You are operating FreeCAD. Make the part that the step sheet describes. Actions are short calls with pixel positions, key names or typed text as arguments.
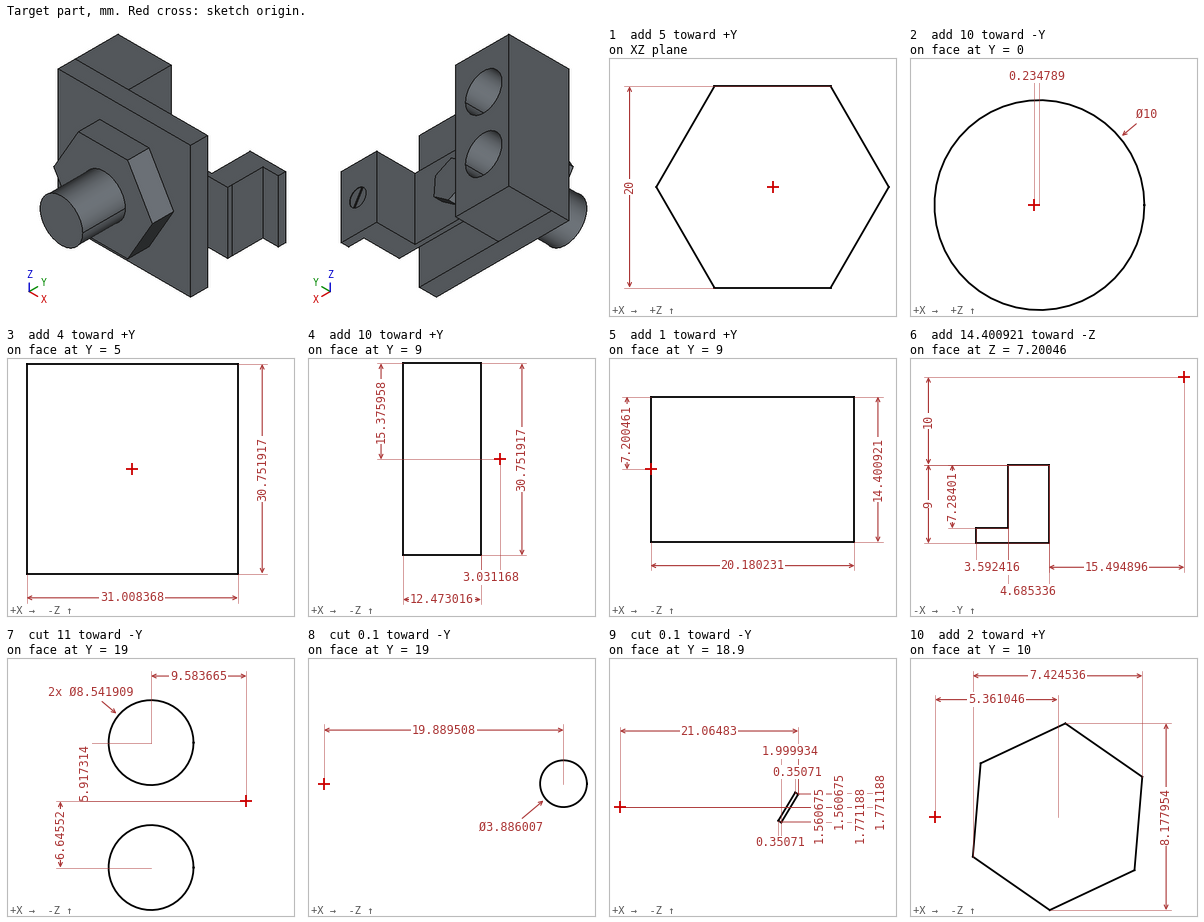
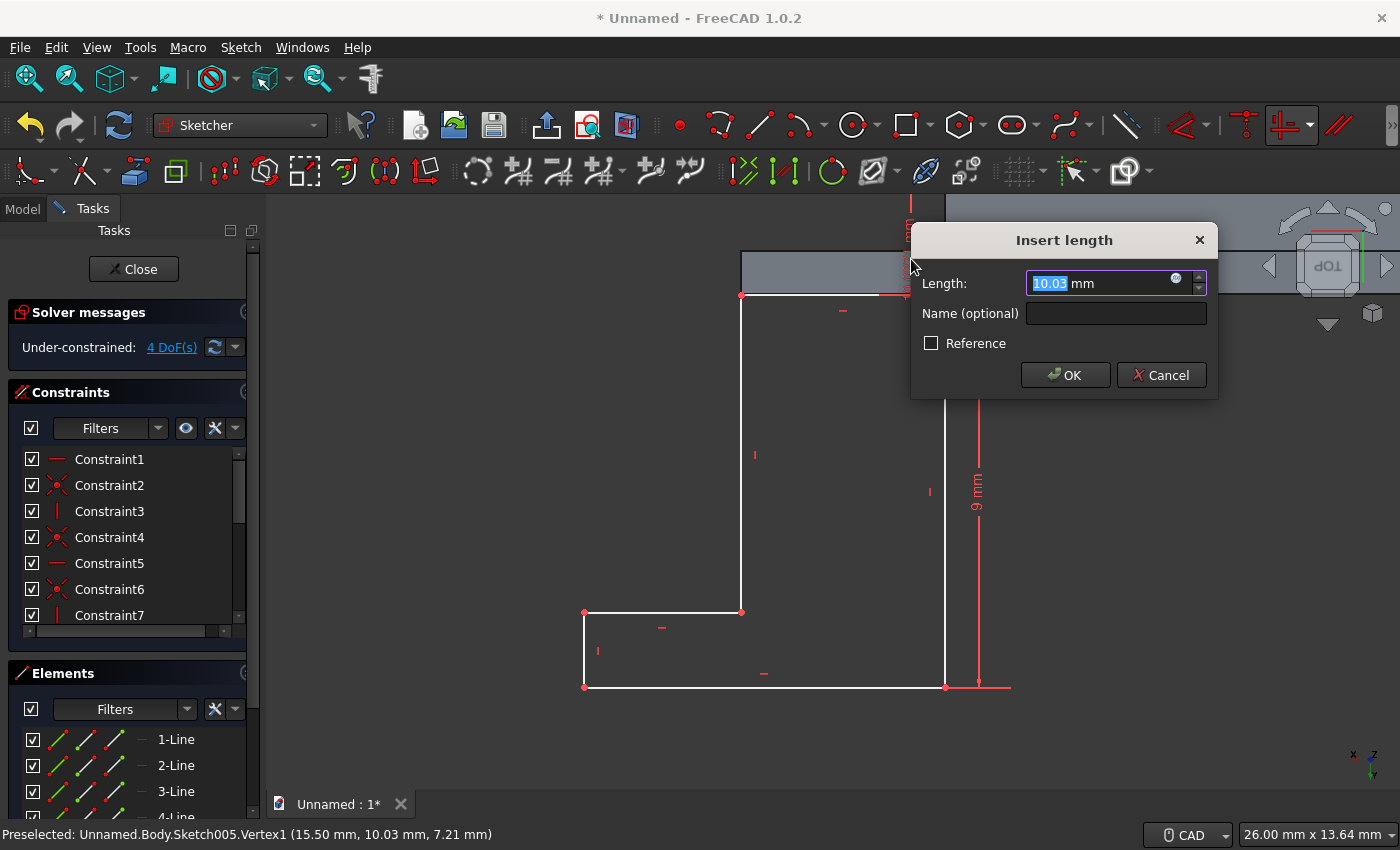
text(10)
key(Return)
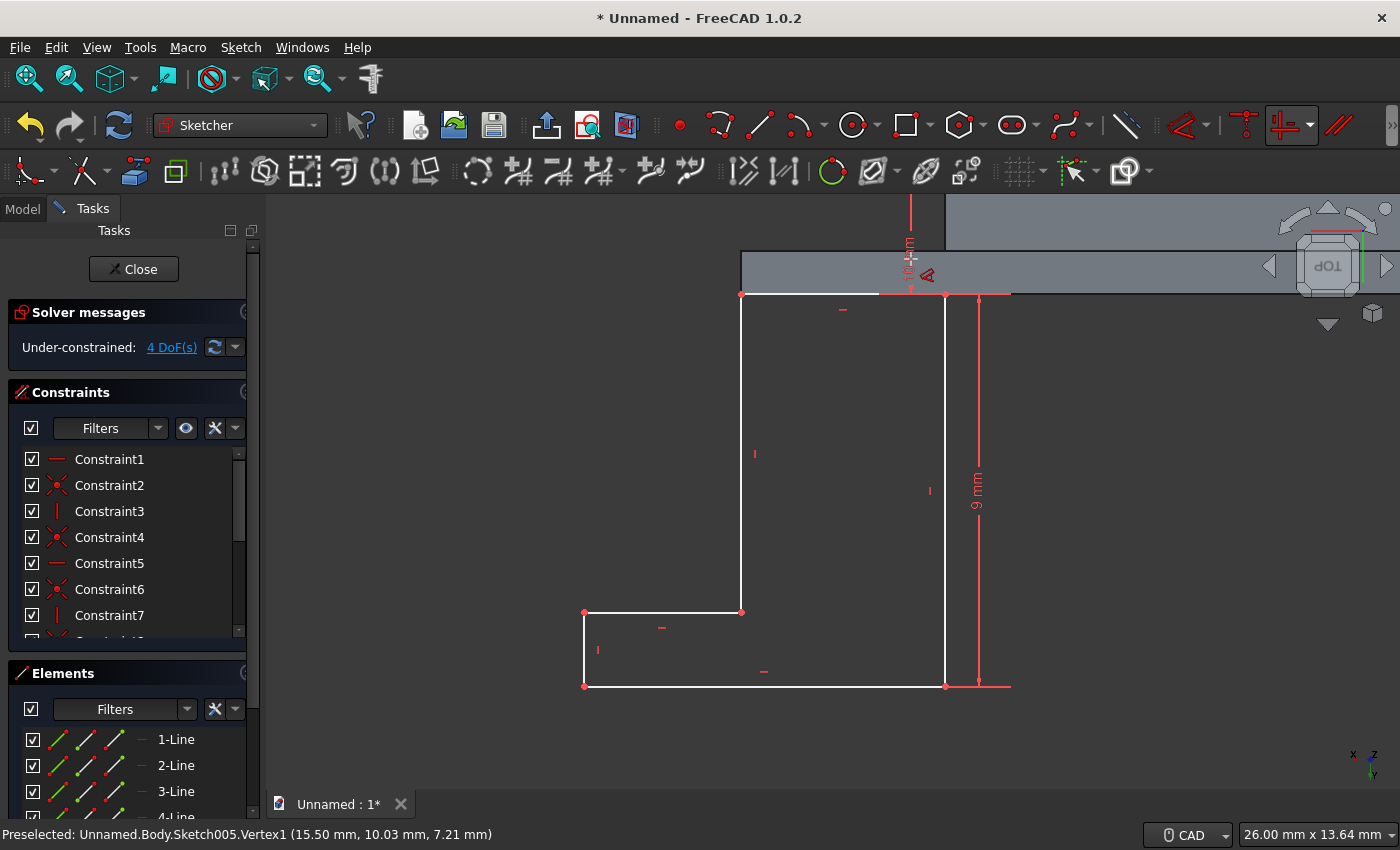
click(741, 390)
click(707, 454)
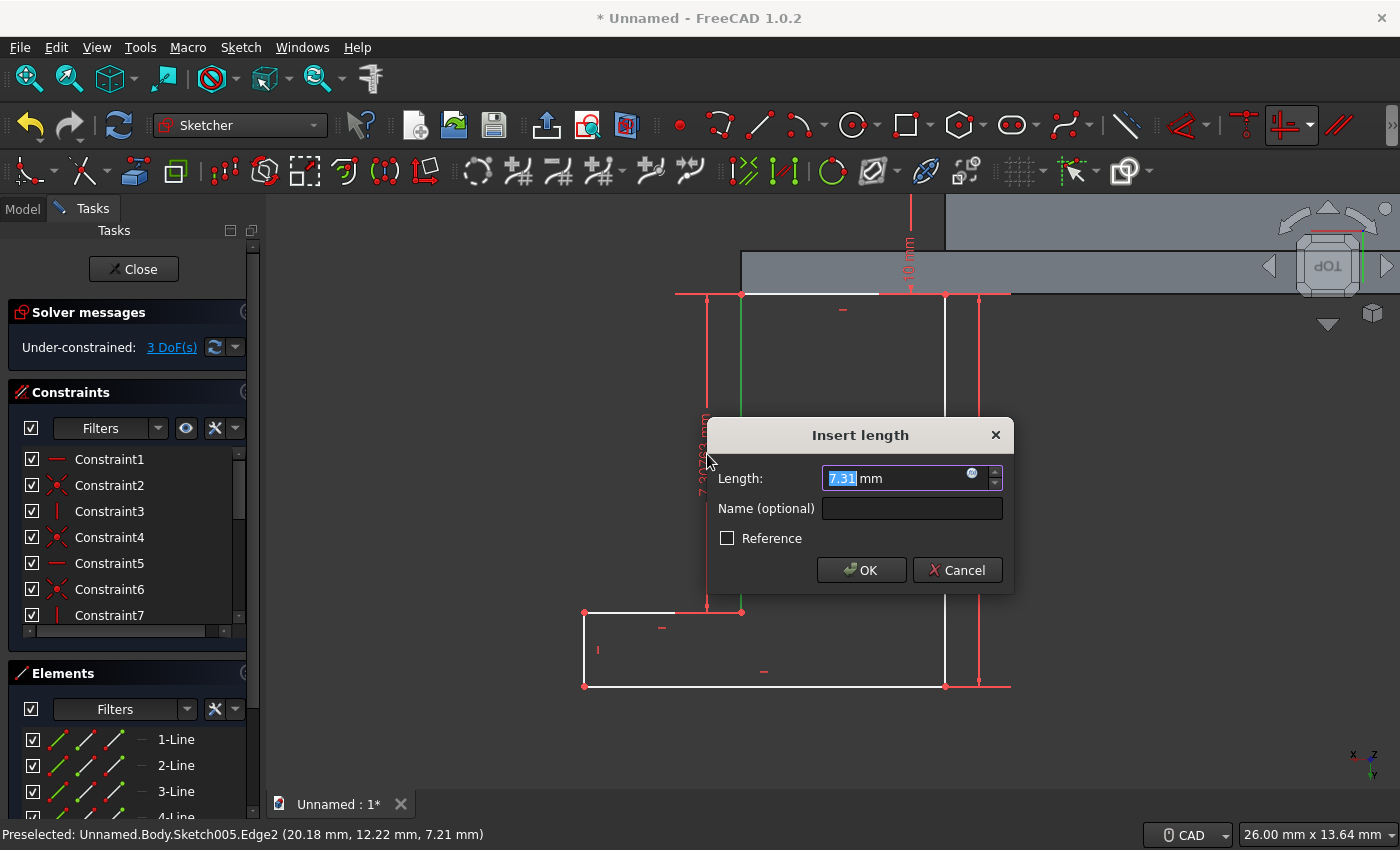
text(7.28401)
key(Return)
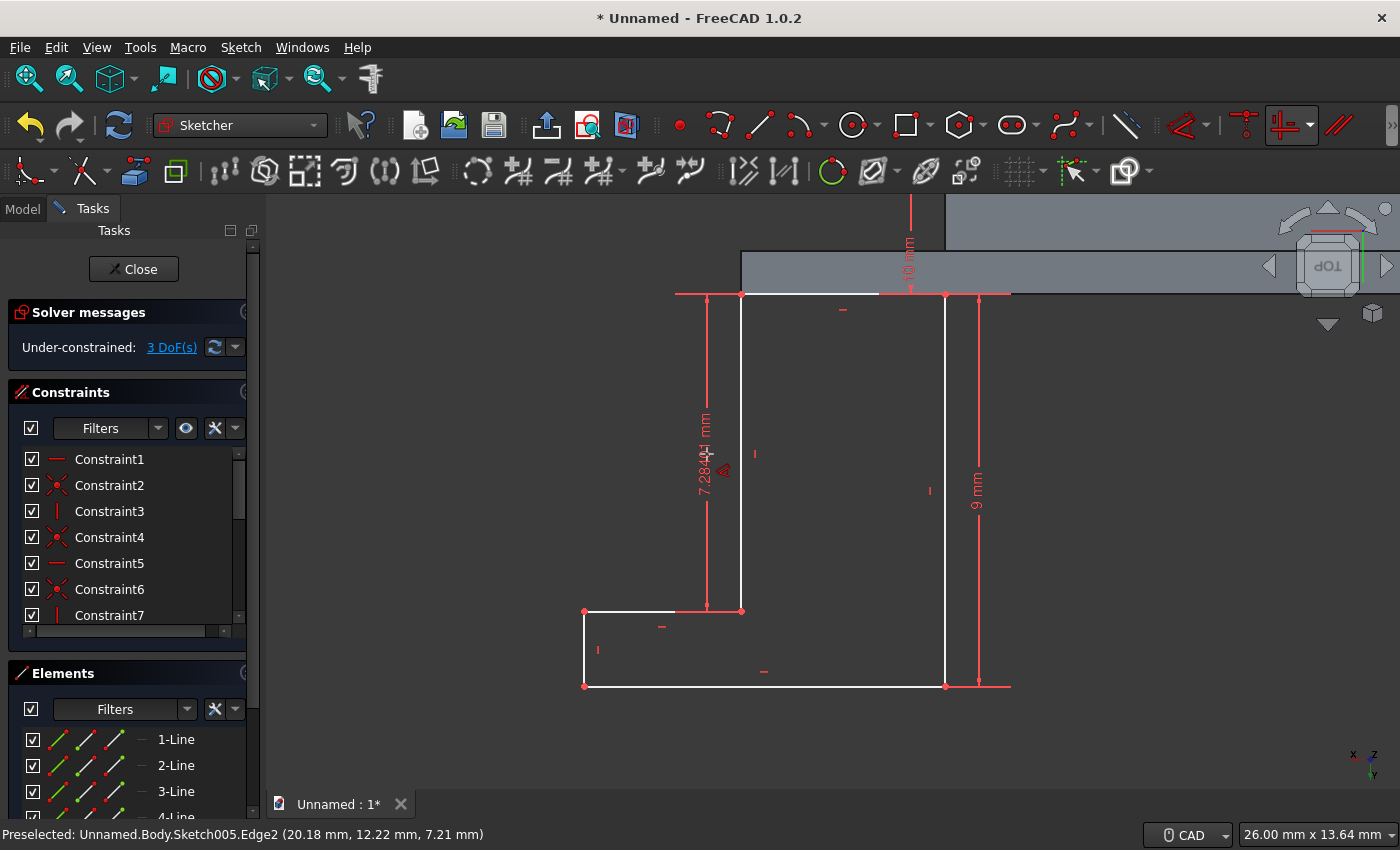
click(884, 294)
click(796, 260)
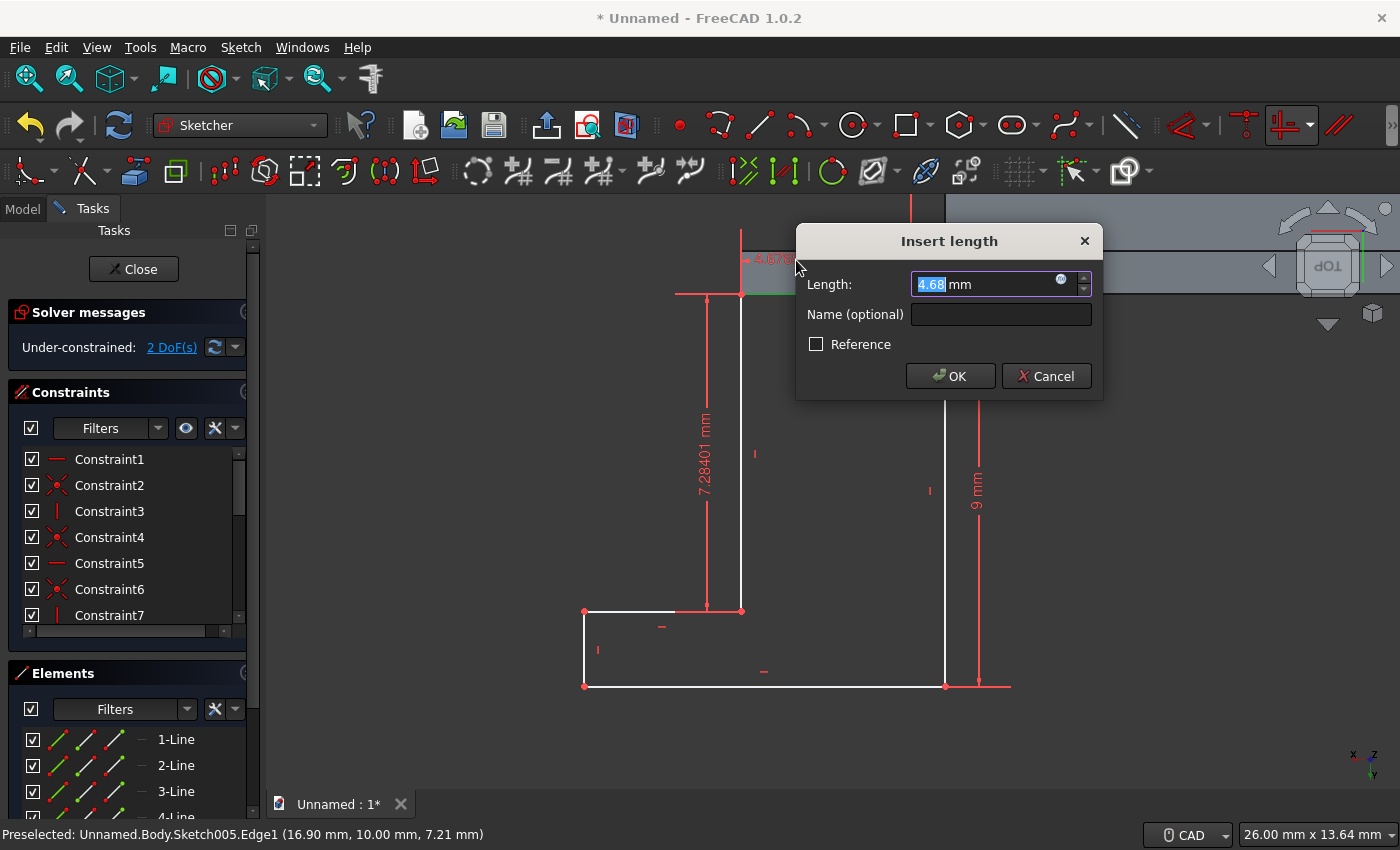
text(4.685336)
key(Return)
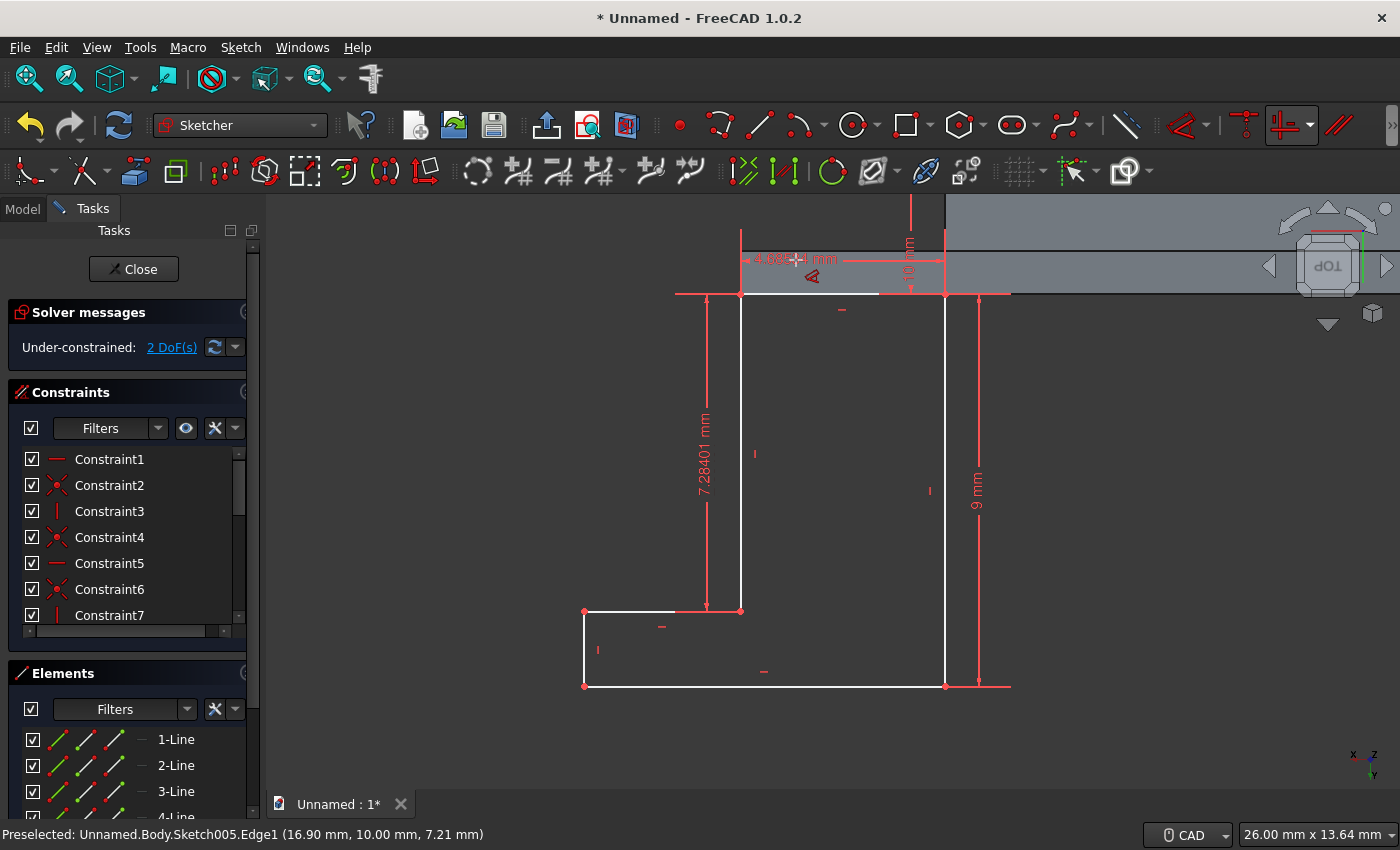
click(694, 612)
click(662, 646)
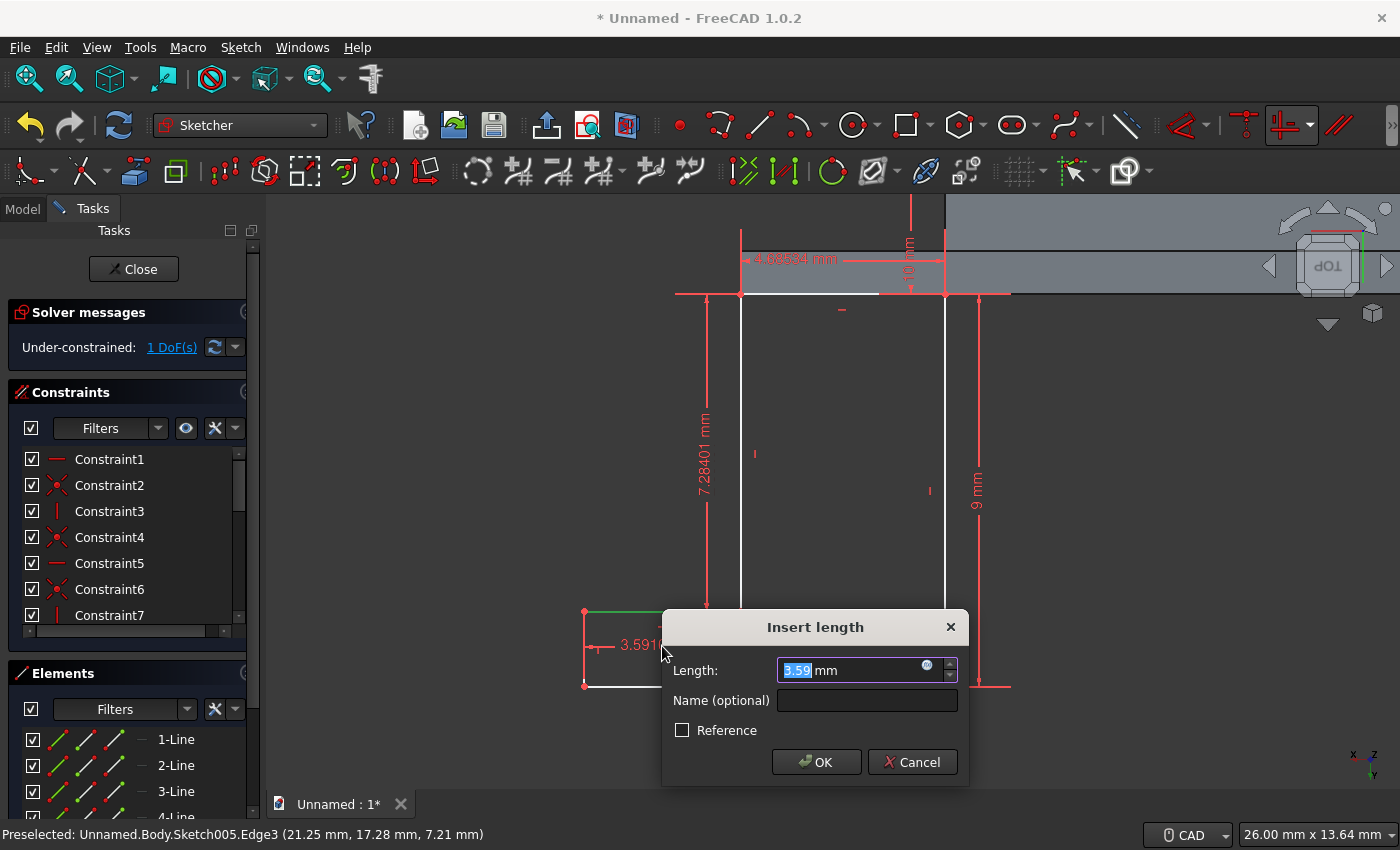
text(3.592416)
key(Return)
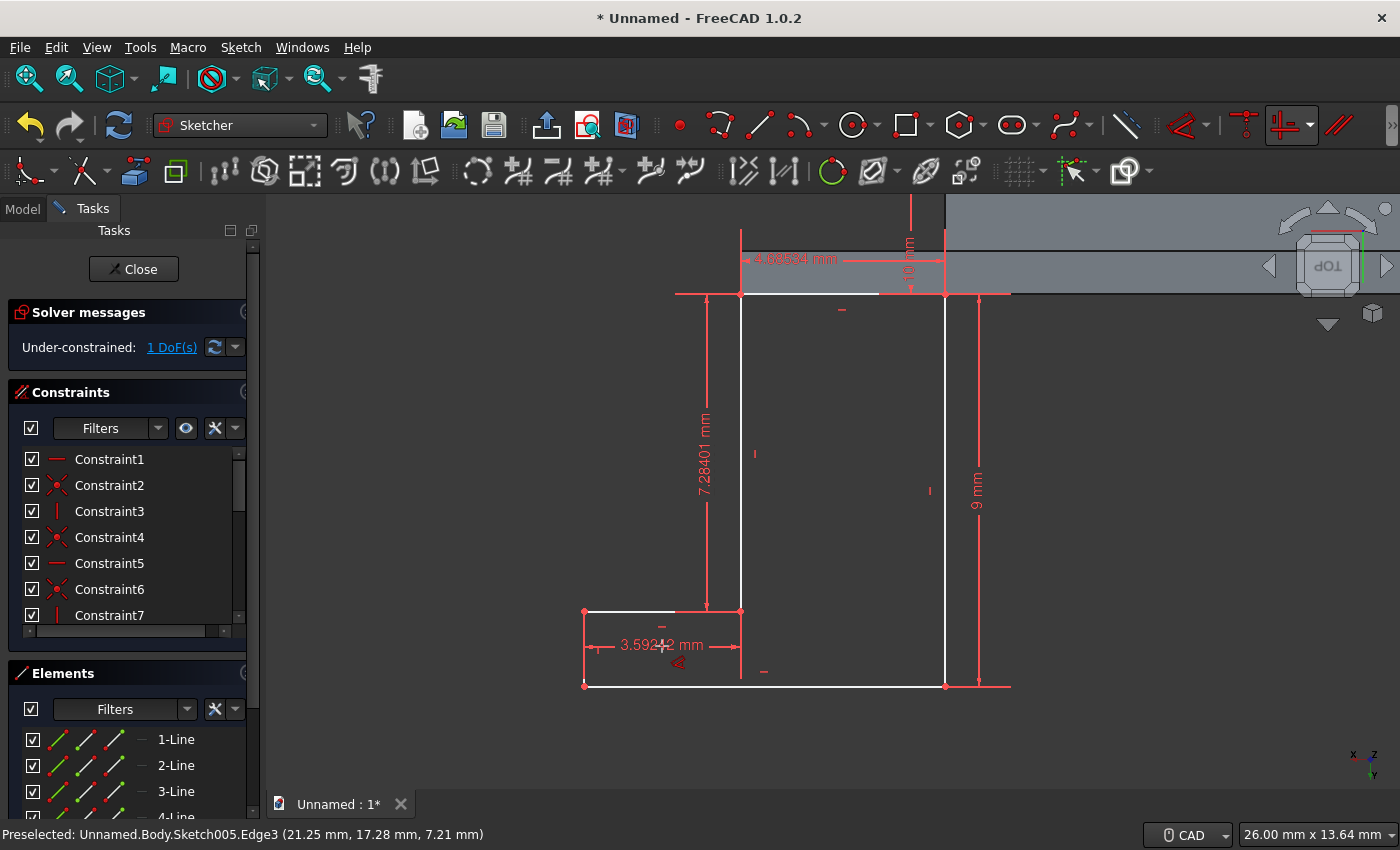
click(945, 294)
click(1090, 328)